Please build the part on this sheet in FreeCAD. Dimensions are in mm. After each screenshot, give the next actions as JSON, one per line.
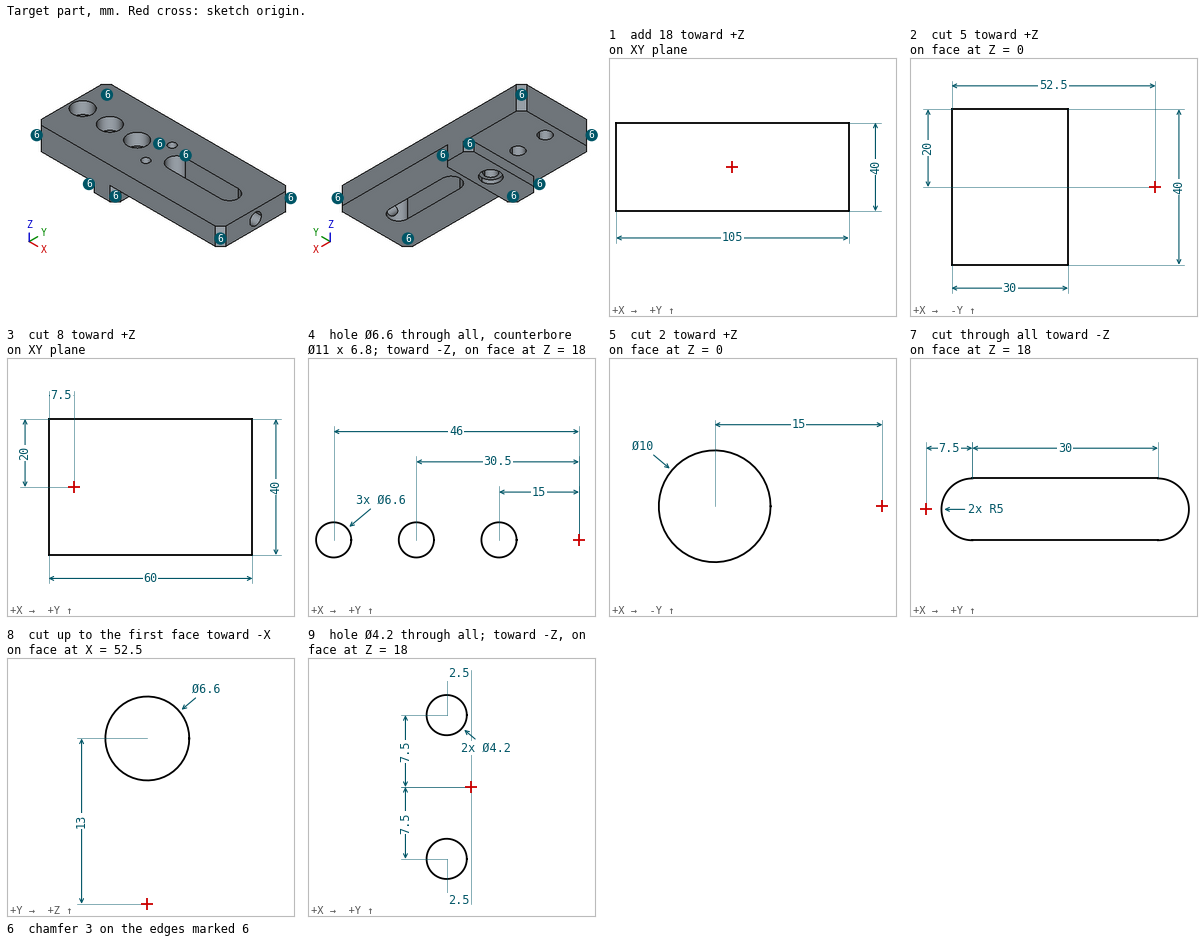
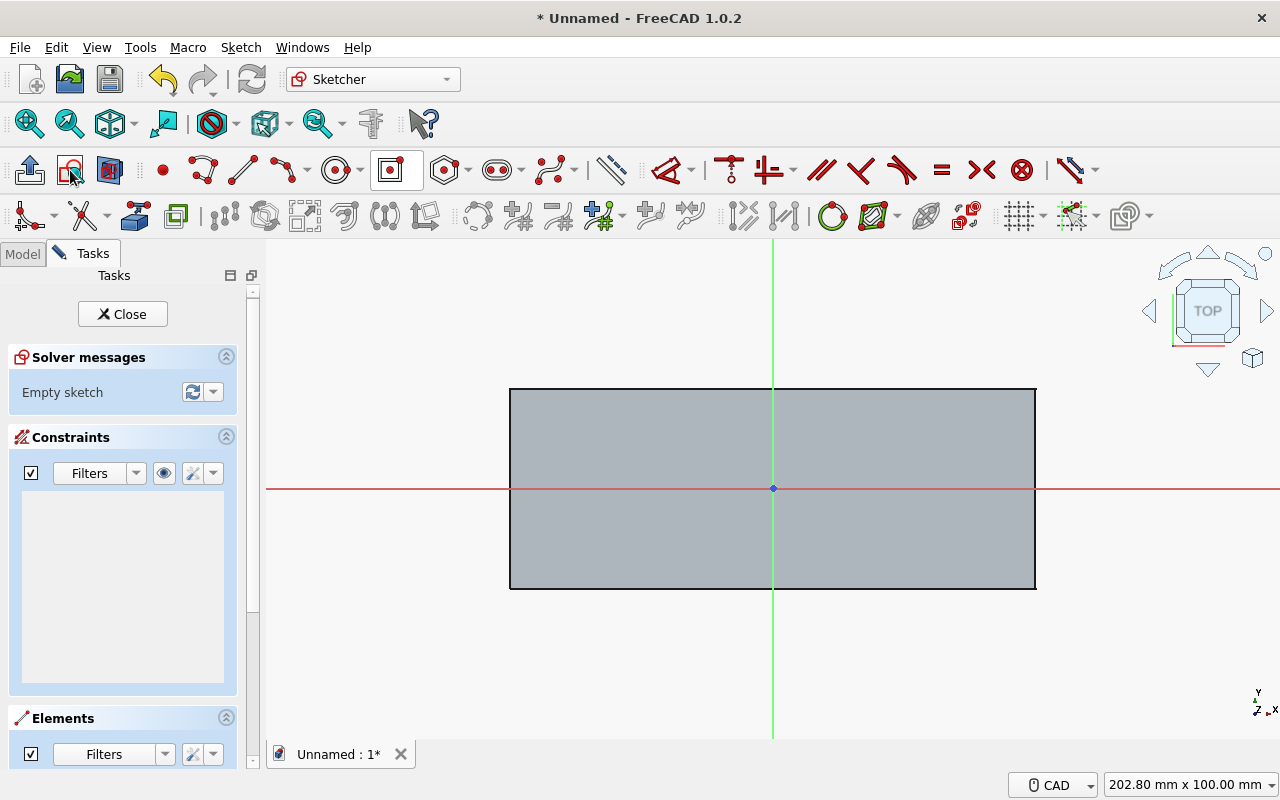
{"action": "scroll", "coordinate": [605, 489], "scroll_direction": "up", "scroll_amount": 4}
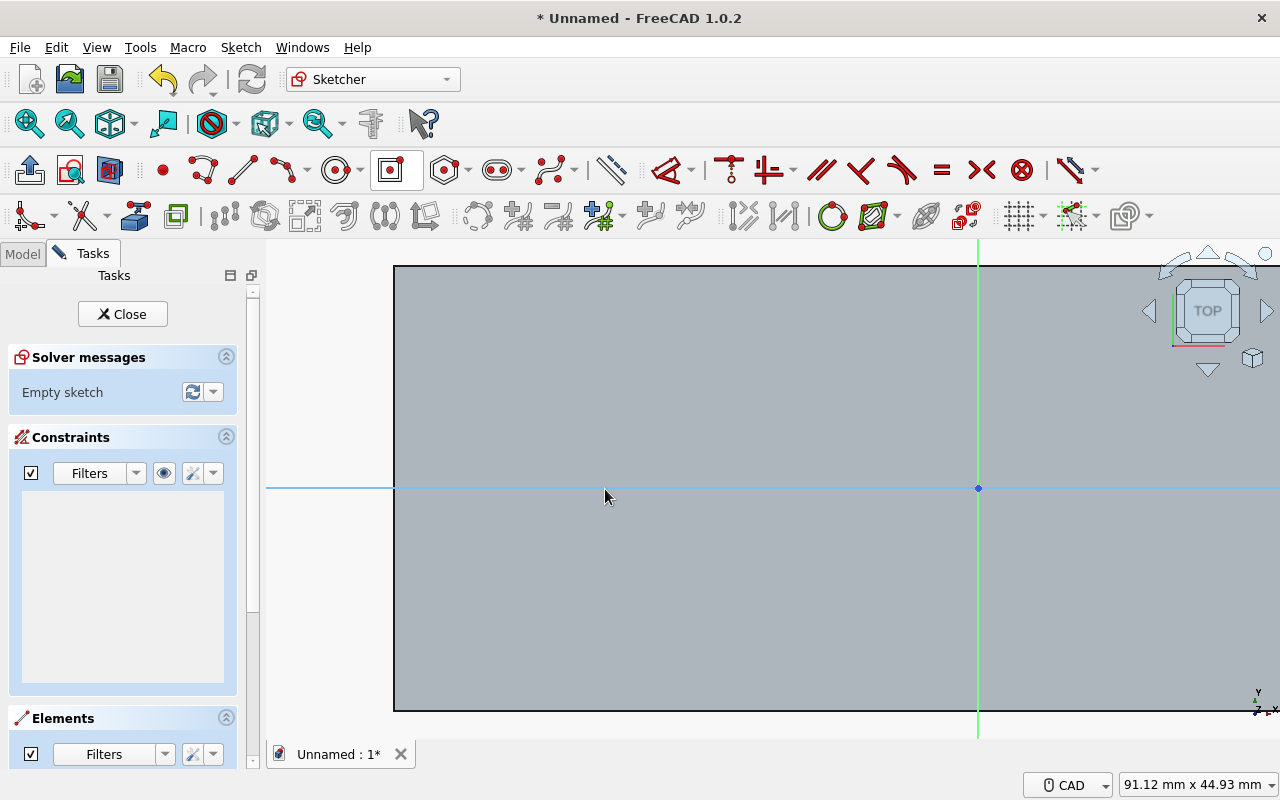
{"action": "key", "text": "g c"}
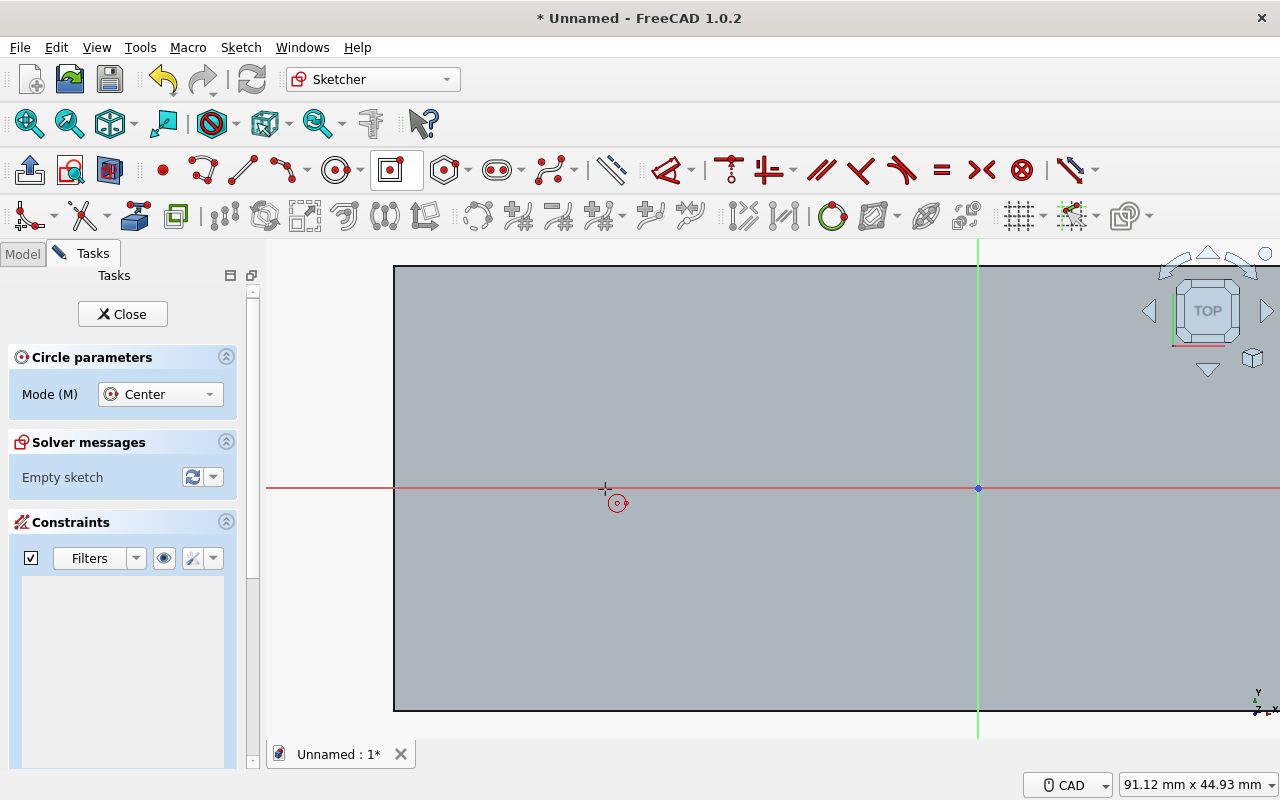
{"action": "left_click", "coordinate": [467, 488]}
{"action": "mouse_move", "coordinate": [493, 462]}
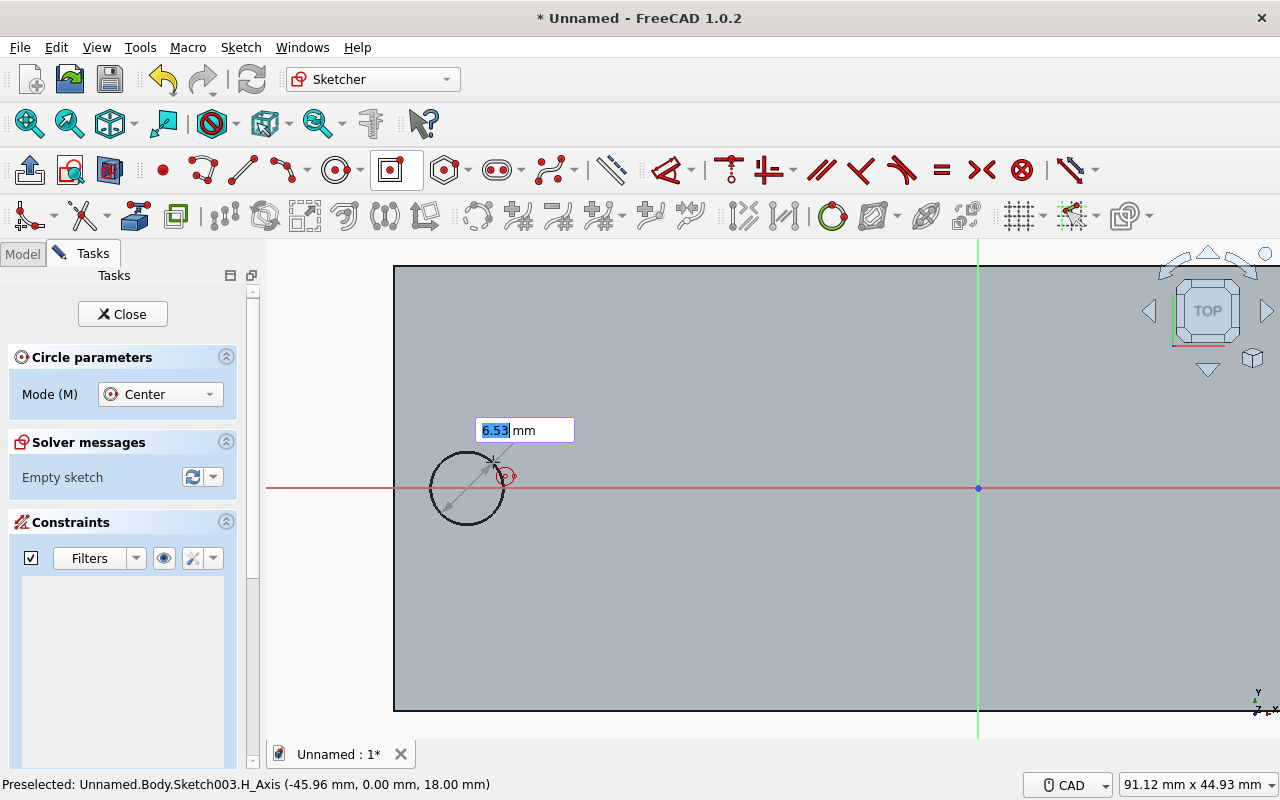
{"action": "type", "text": "6.6"}
{"action": "key", "text": "Return"}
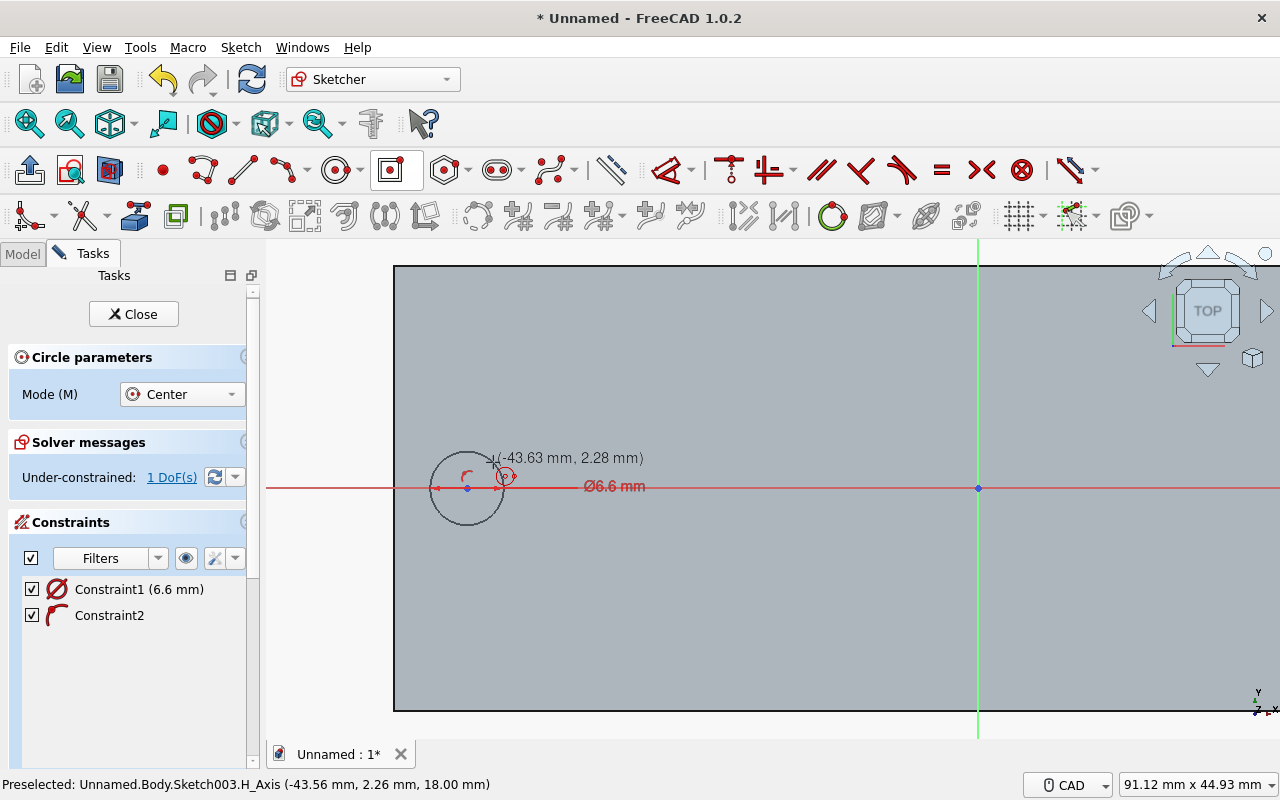
{"action": "left_click", "coordinate": [639, 488]}
{"action": "mouse_move", "coordinate": [665, 462]}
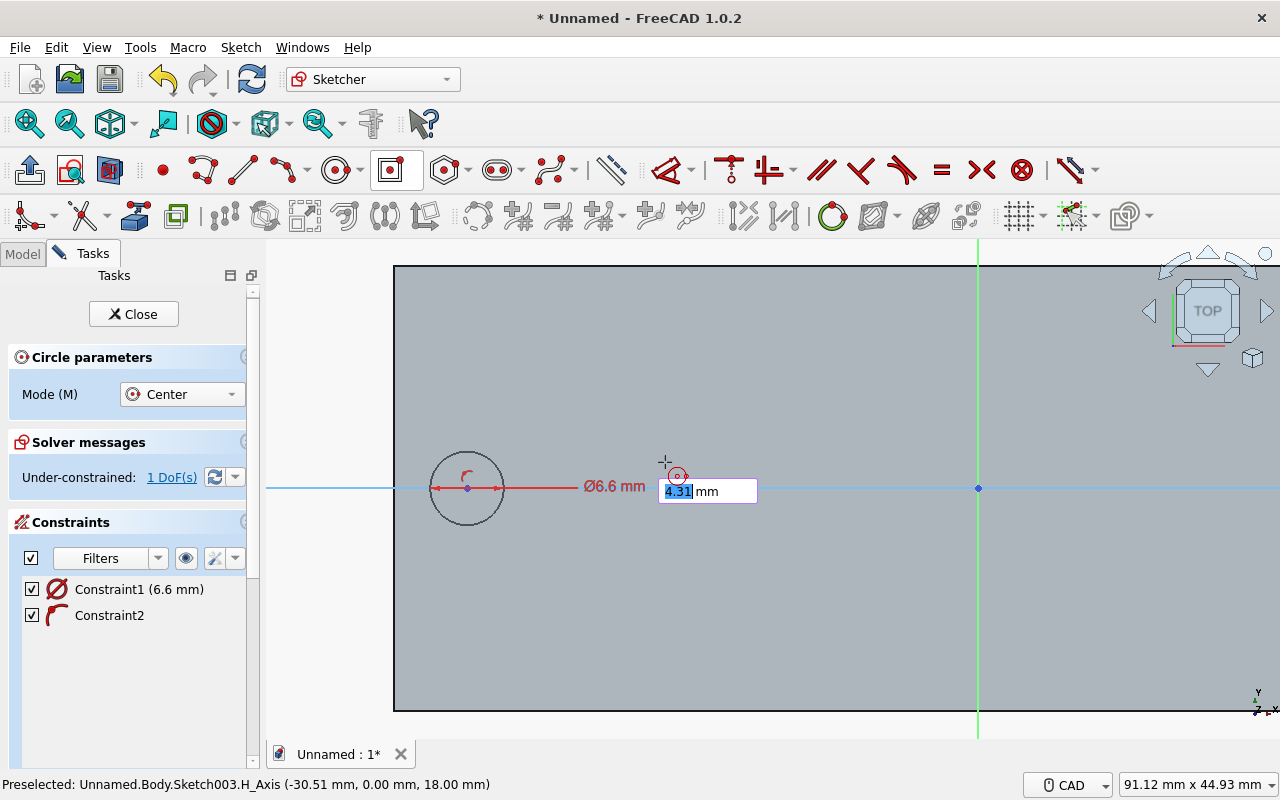
{"action": "type", "text": "6.6"}
{"action": "key", "text": "Return"}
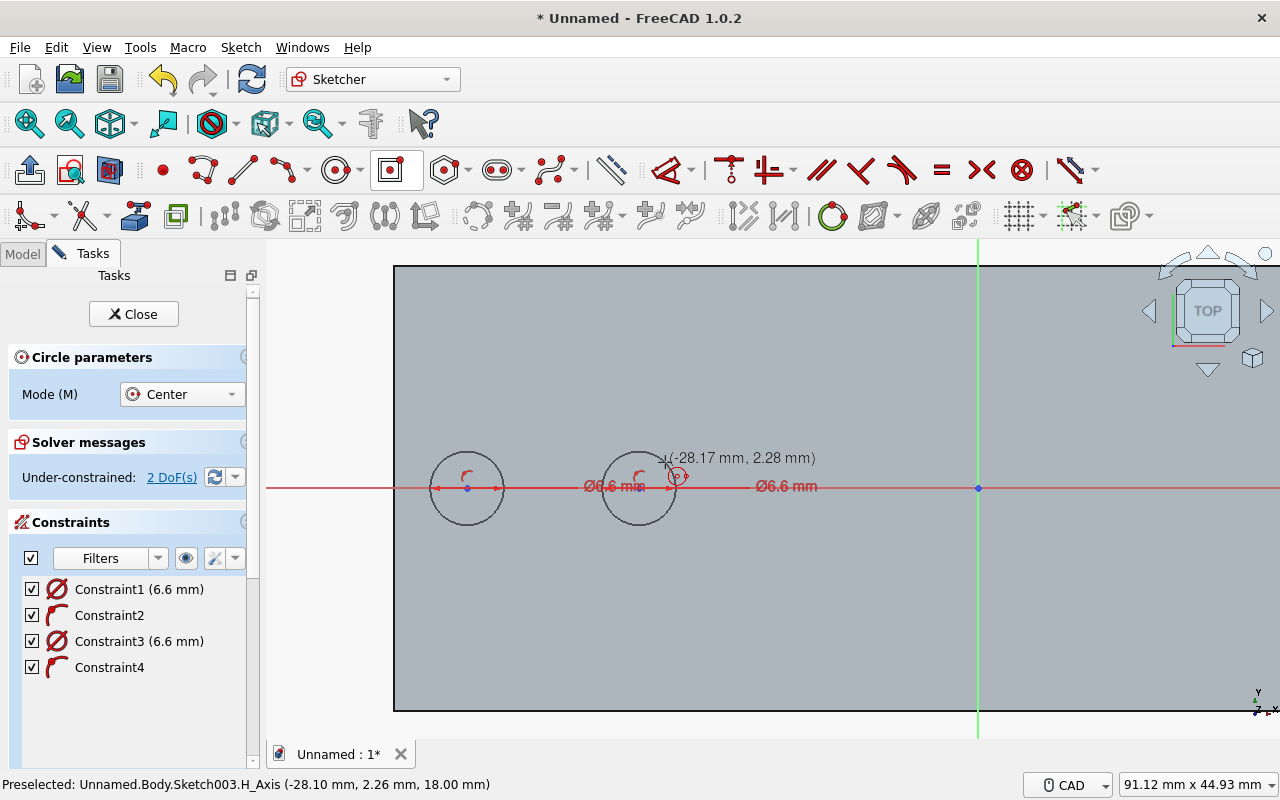
{"action": "left_click", "coordinate": [812, 488]}
{"action": "mouse_move", "coordinate": [838, 462]}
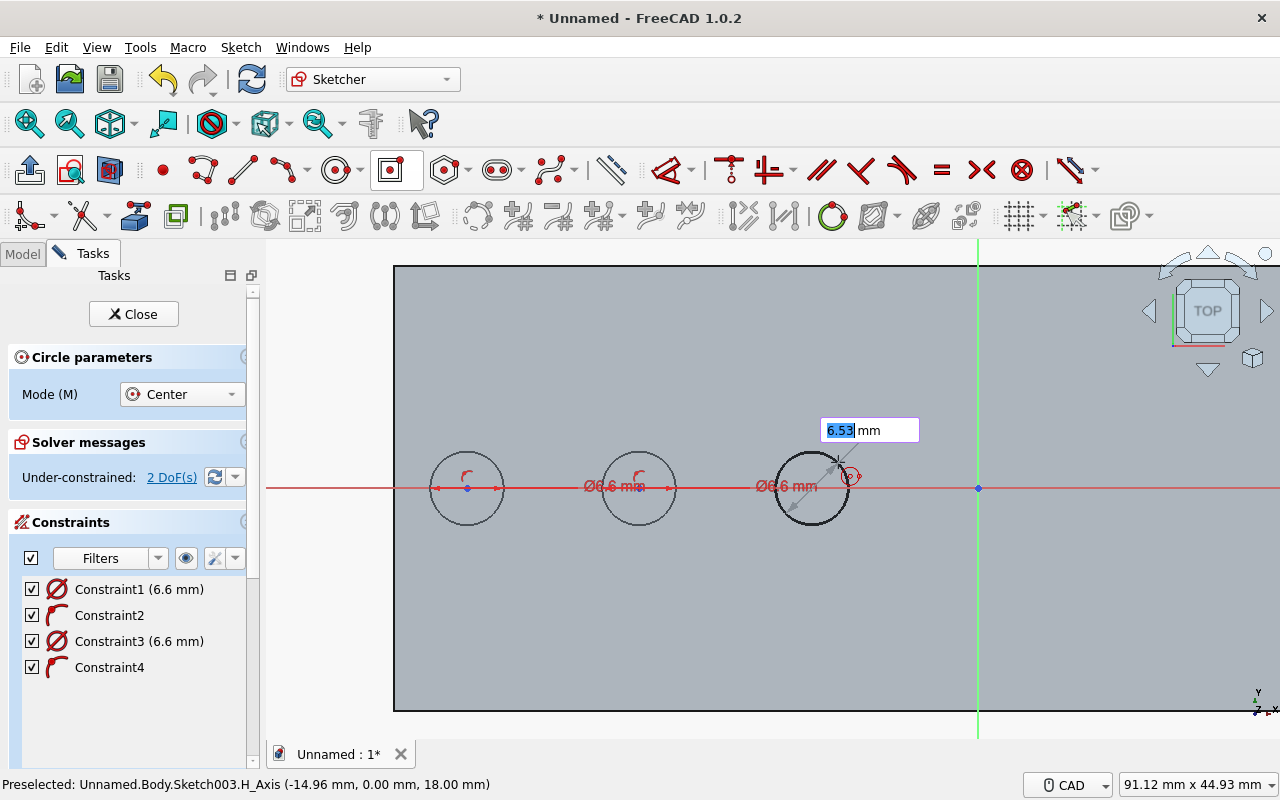
{"action": "type", "text": "6.6"}
{"action": "key", "text": "Return"}
{"action": "key", "text": "Escape"}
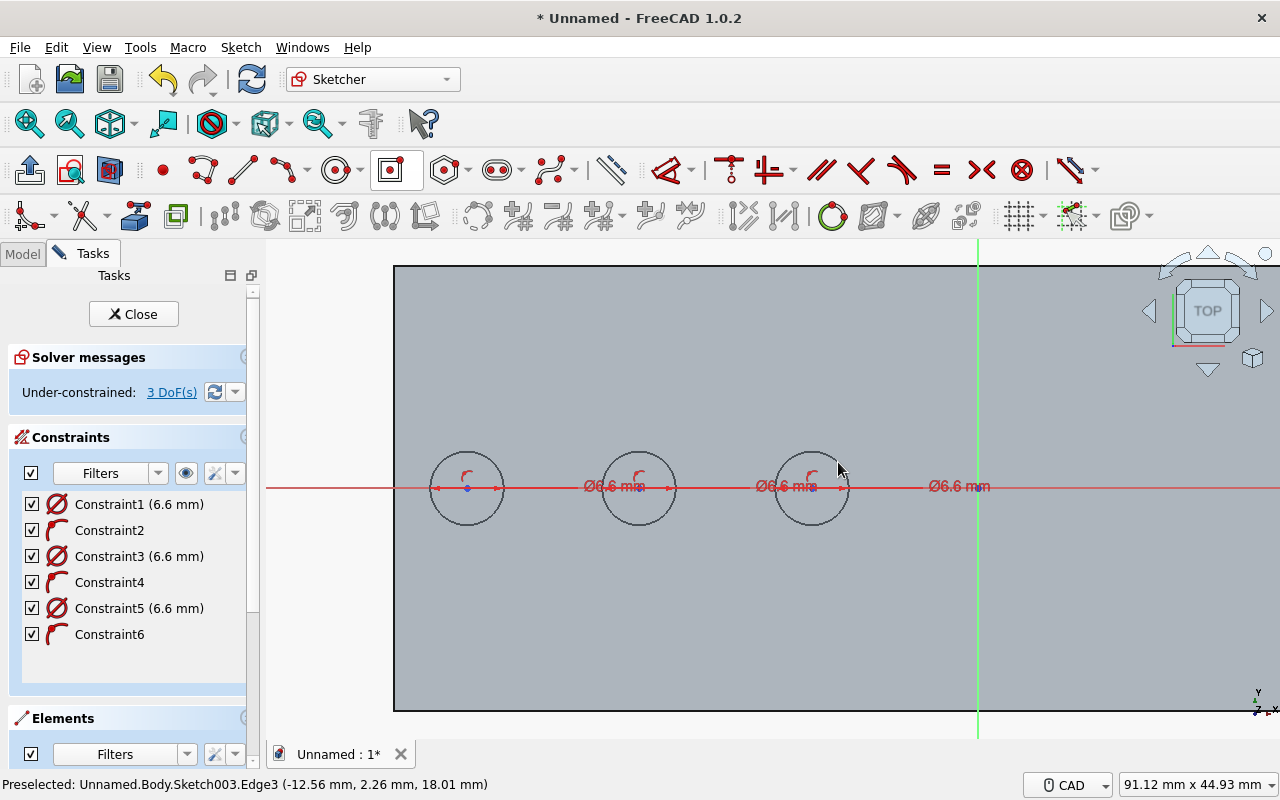
{"action": "left_click", "coordinate": [666, 170]}